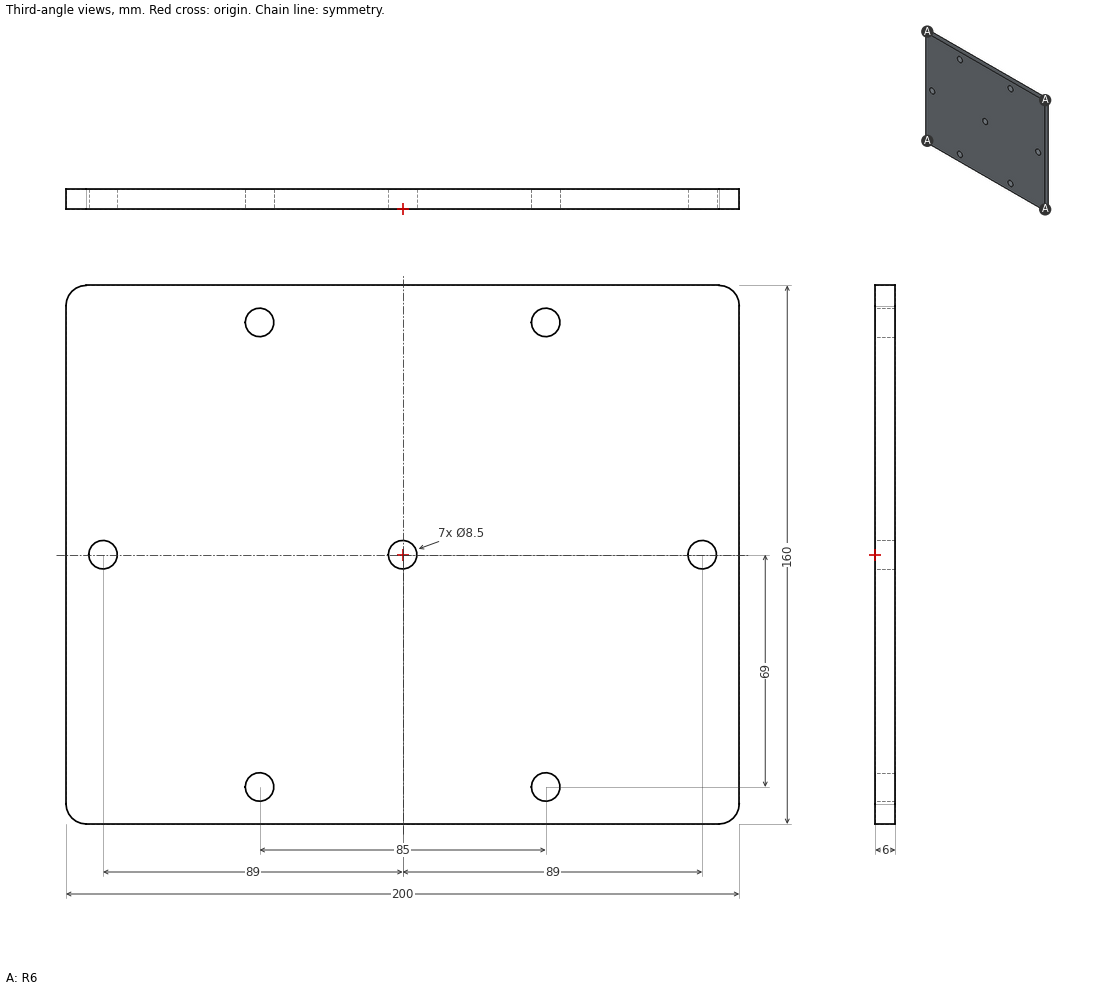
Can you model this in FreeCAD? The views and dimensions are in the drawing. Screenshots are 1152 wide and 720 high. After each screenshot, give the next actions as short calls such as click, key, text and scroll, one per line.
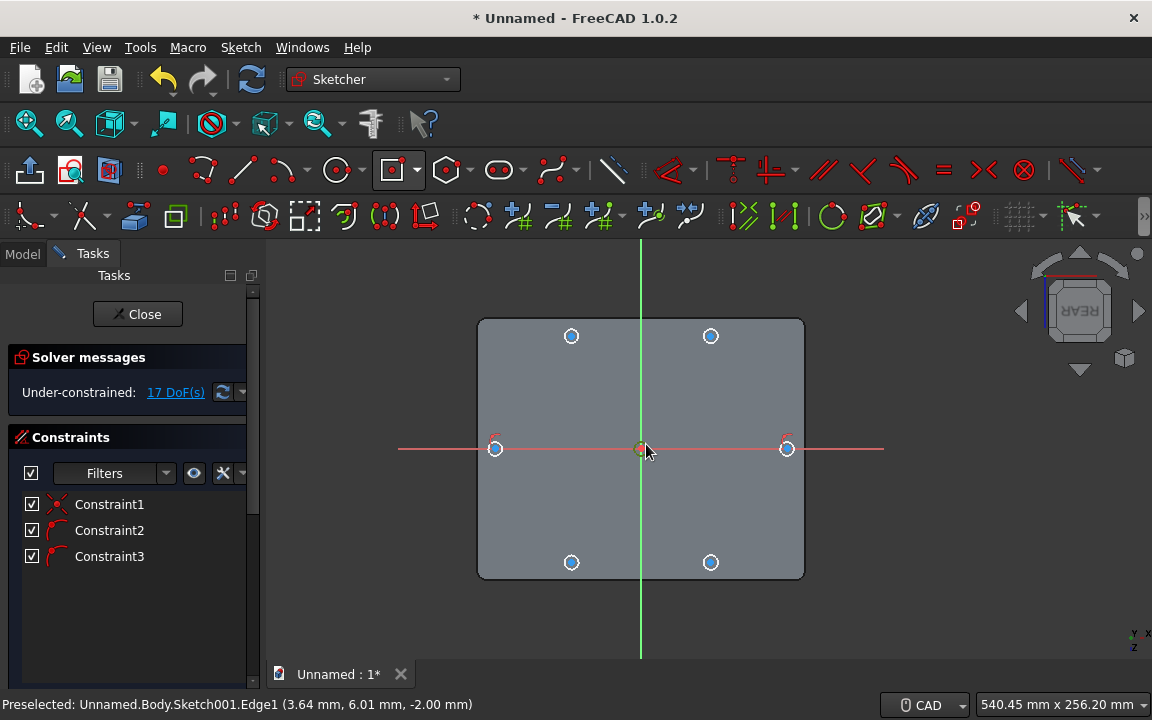
scroll(716, 331, up, 4)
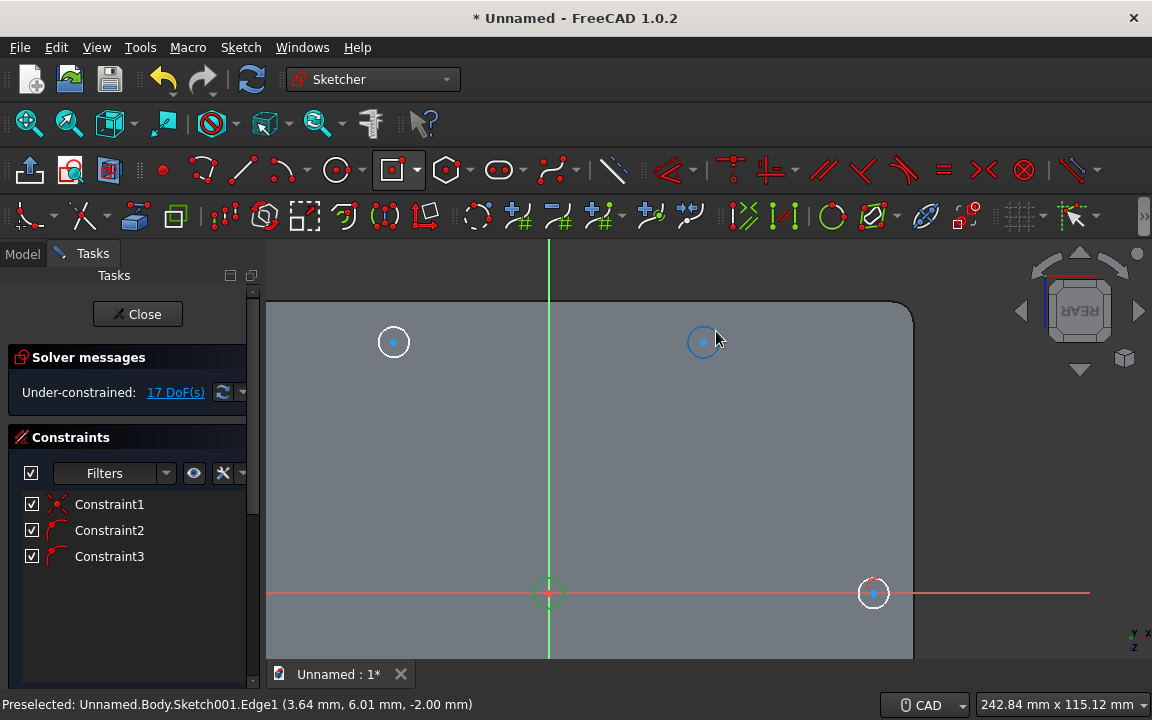
click(715, 331)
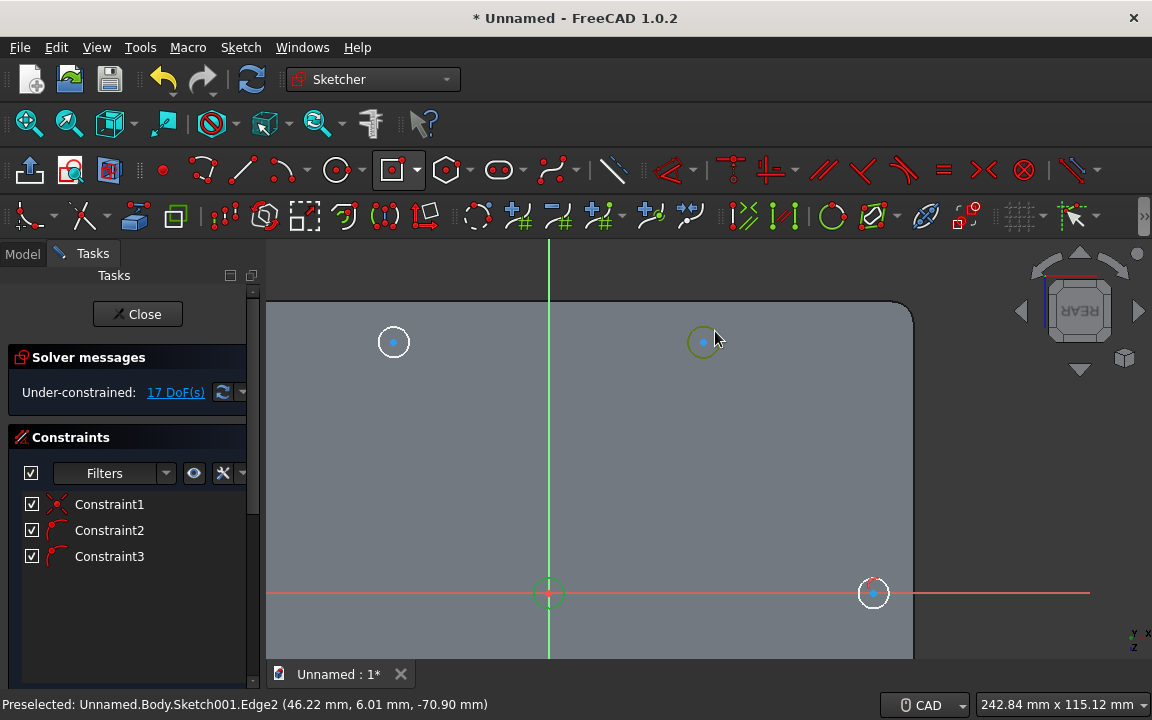
click(405, 331)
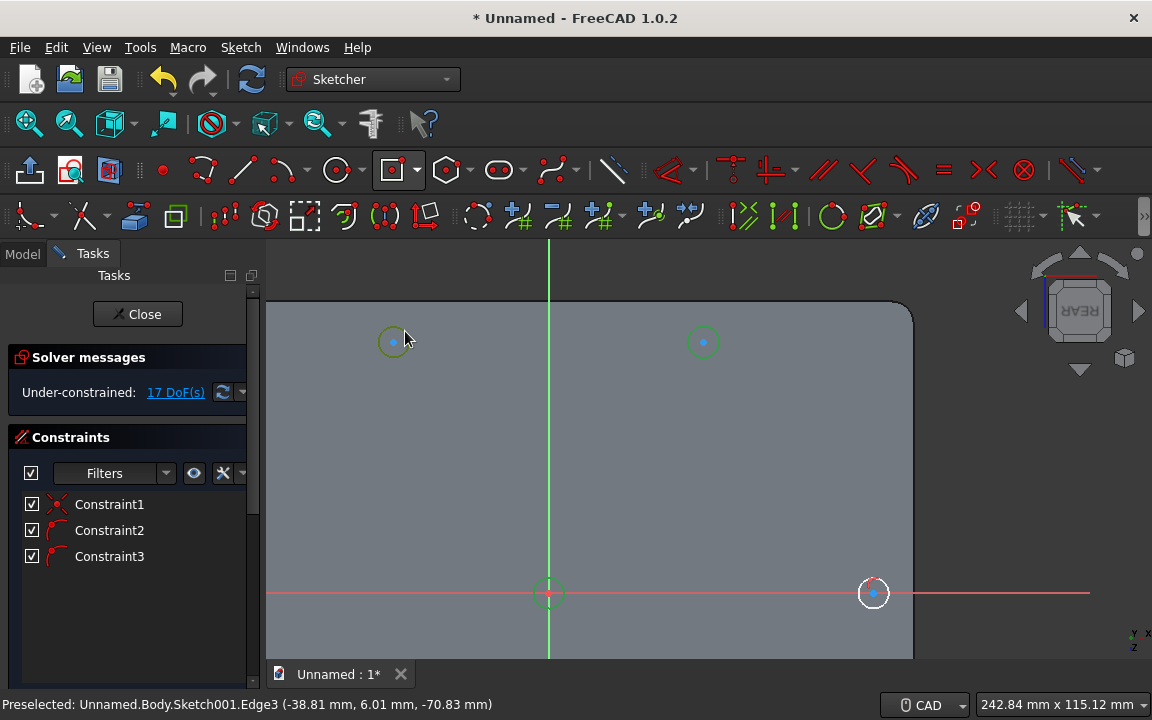
scroll(715, 331, down, 4)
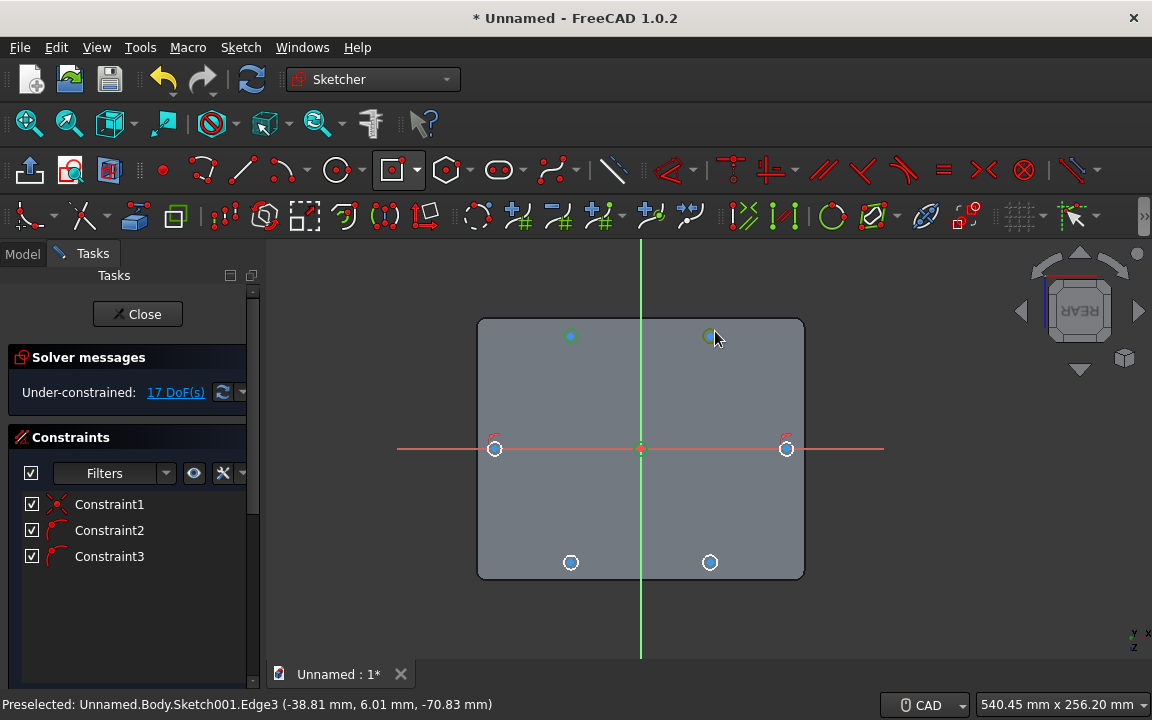
scroll(500, 444, up, 6)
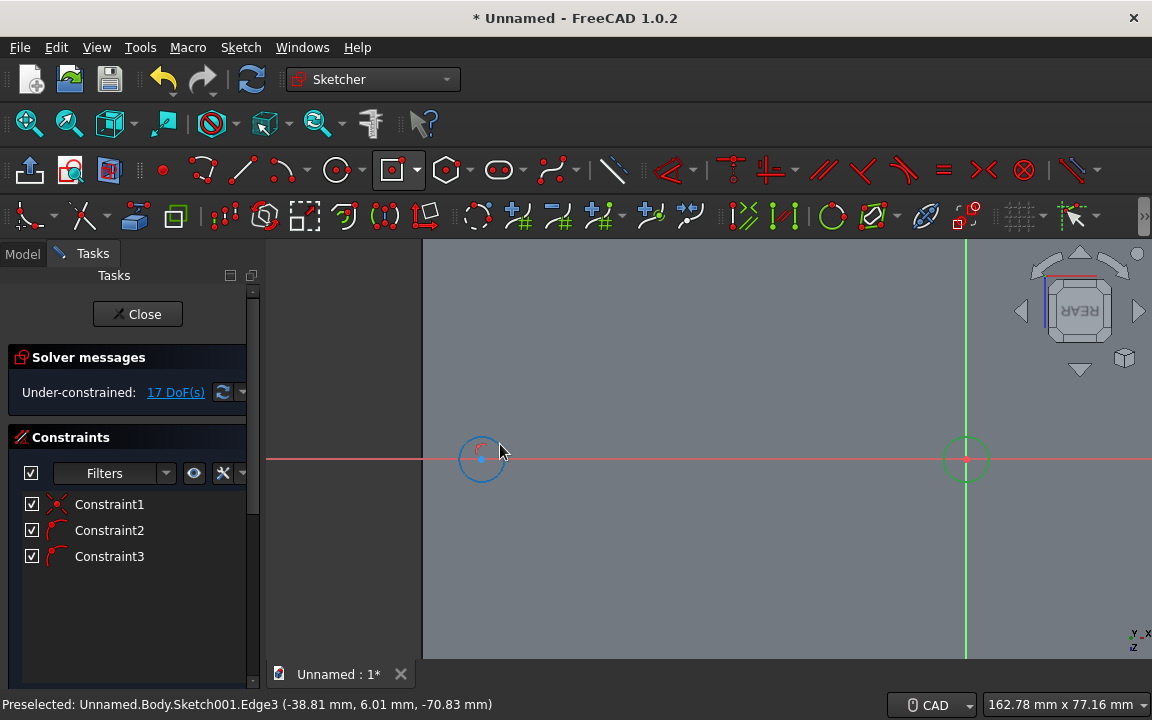
click(498, 443)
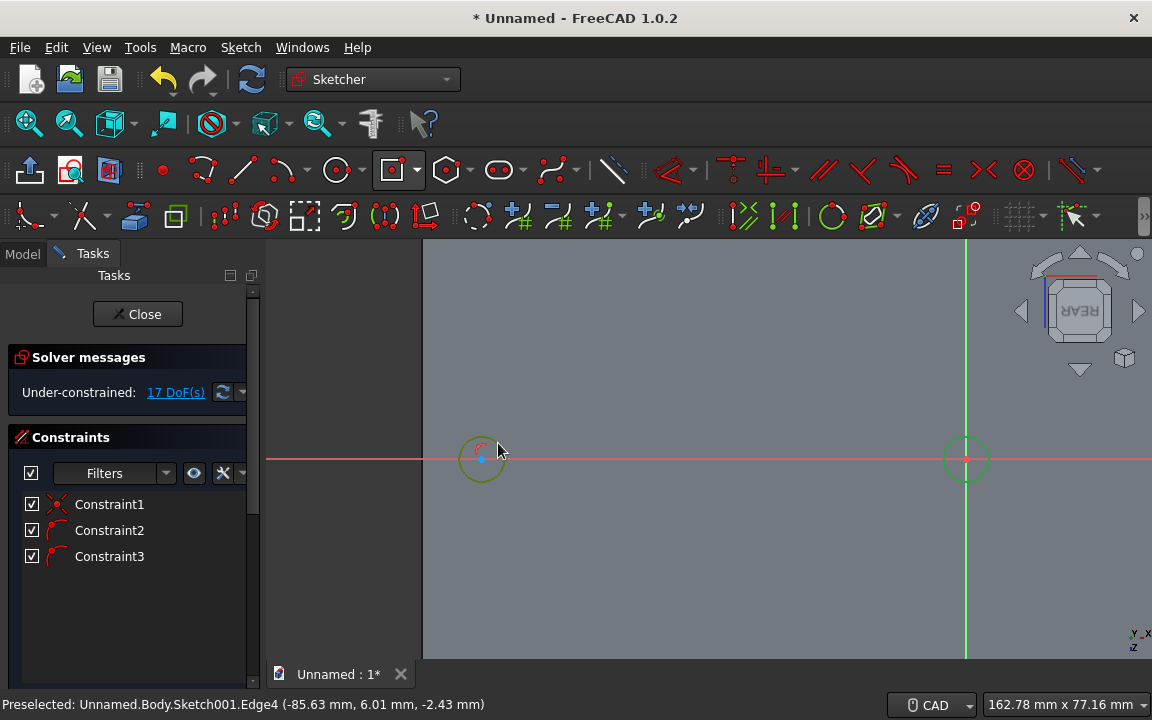
scroll(500, 444, down, 6)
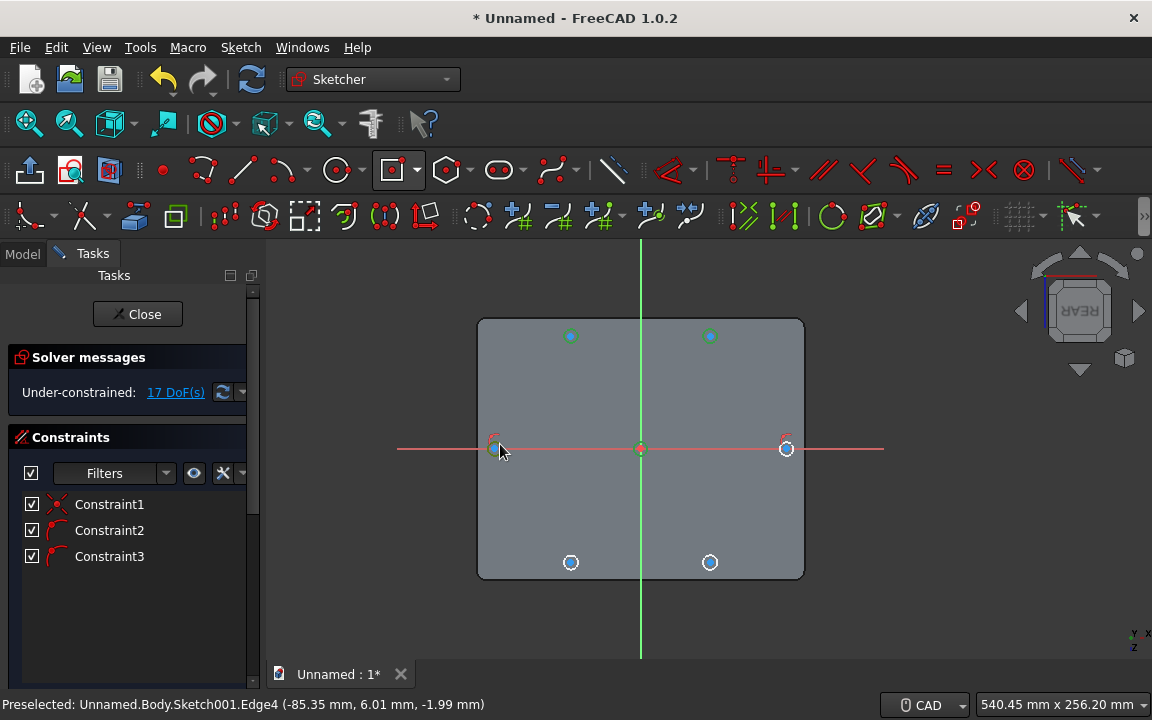
scroll(791, 444, up, 6)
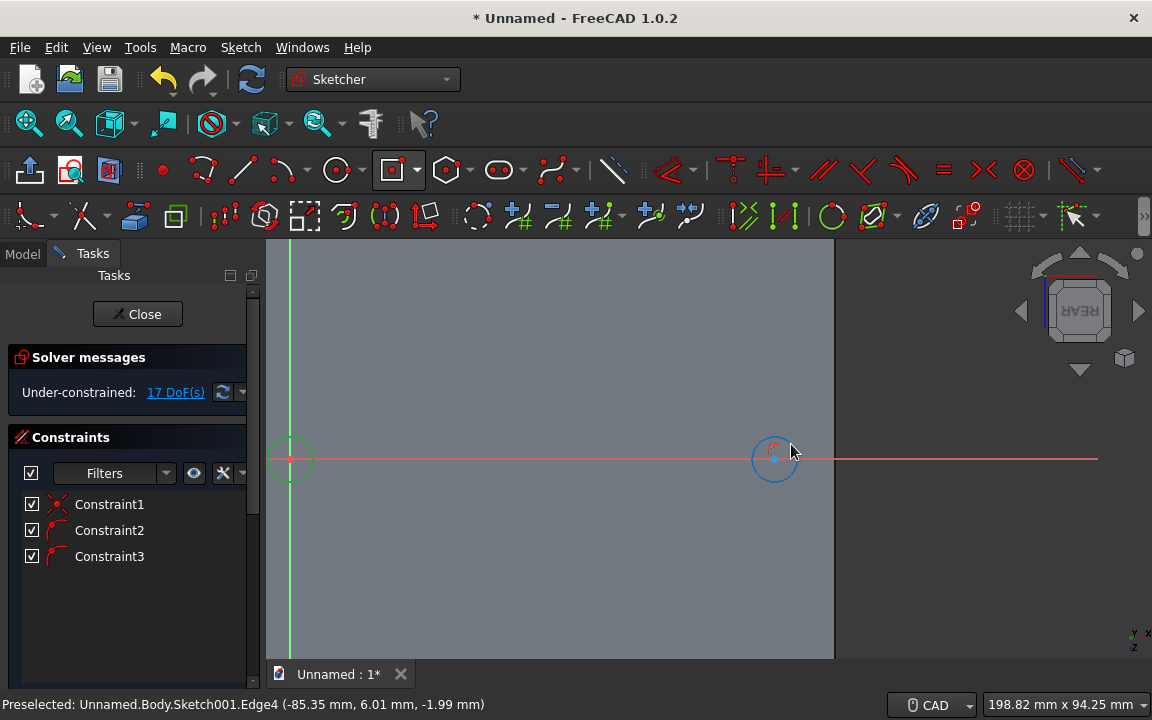
click(791, 443)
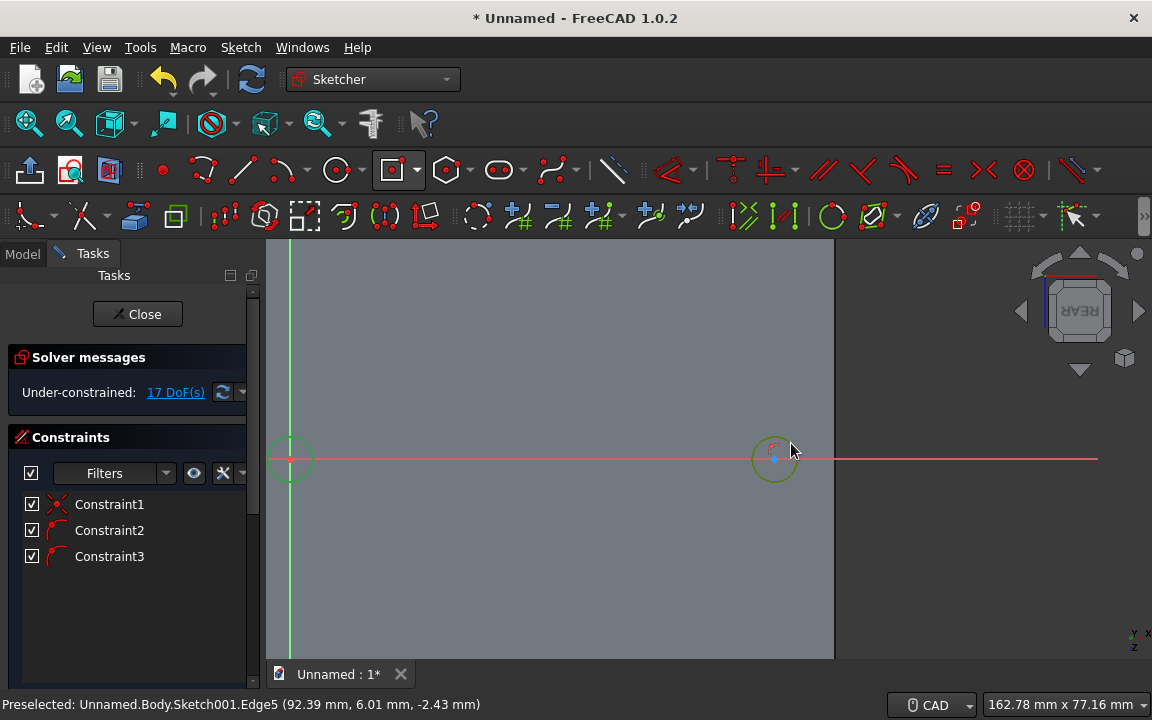
scroll(791, 444, down, 6)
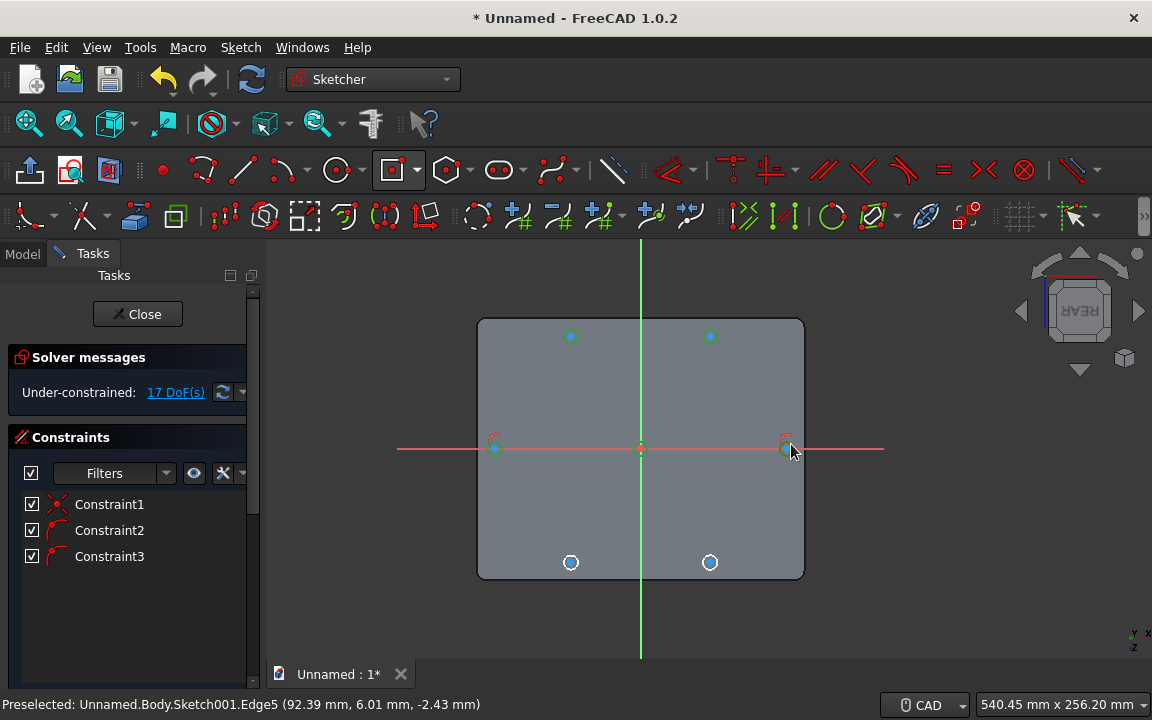
scroll(715, 557, up, 4)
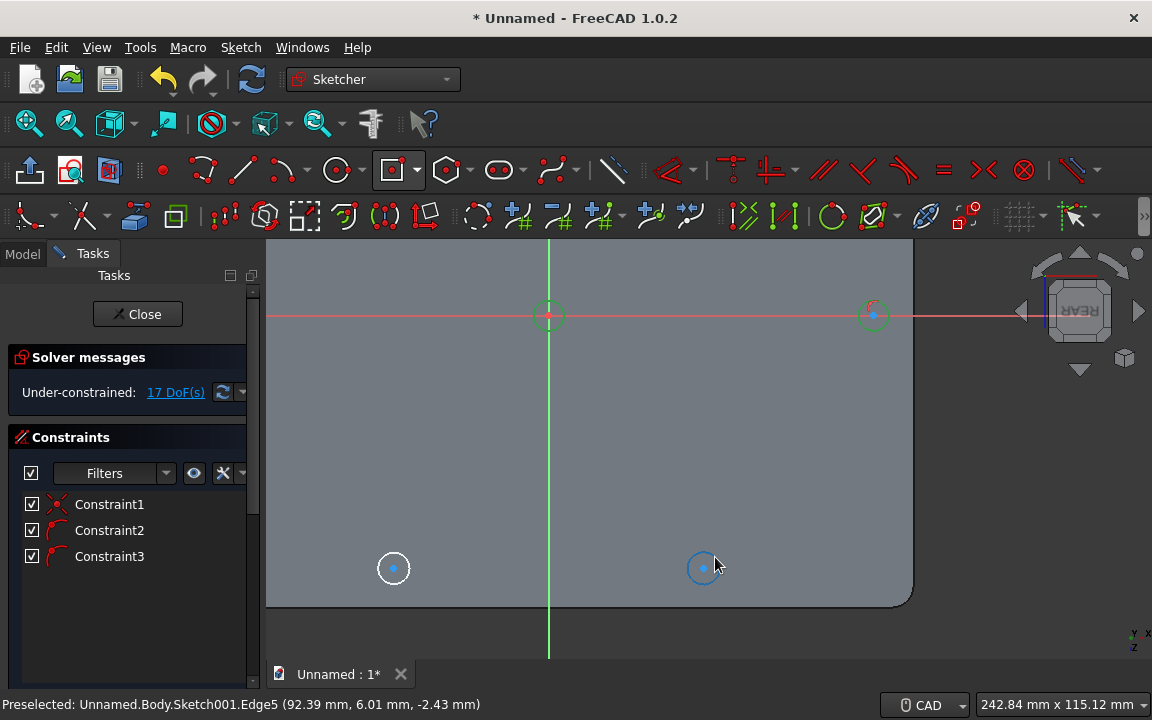
click(715, 557)